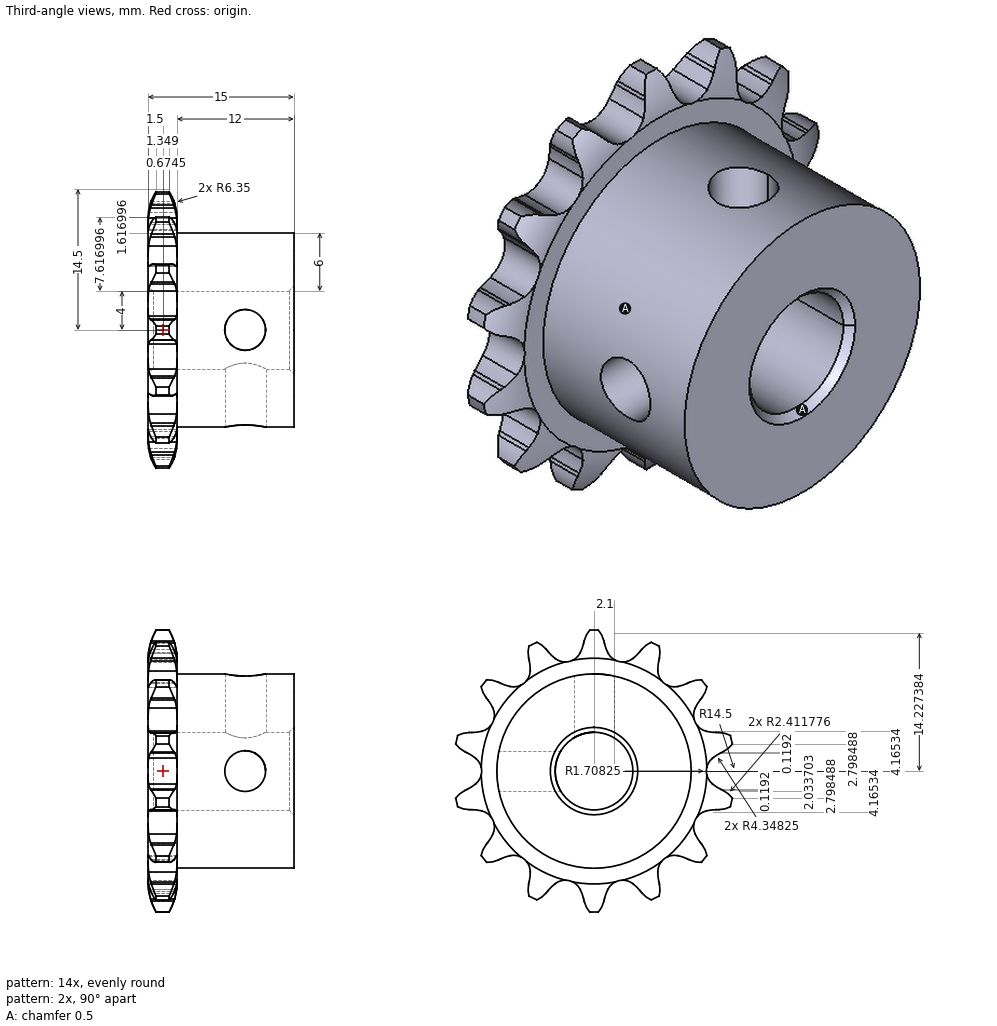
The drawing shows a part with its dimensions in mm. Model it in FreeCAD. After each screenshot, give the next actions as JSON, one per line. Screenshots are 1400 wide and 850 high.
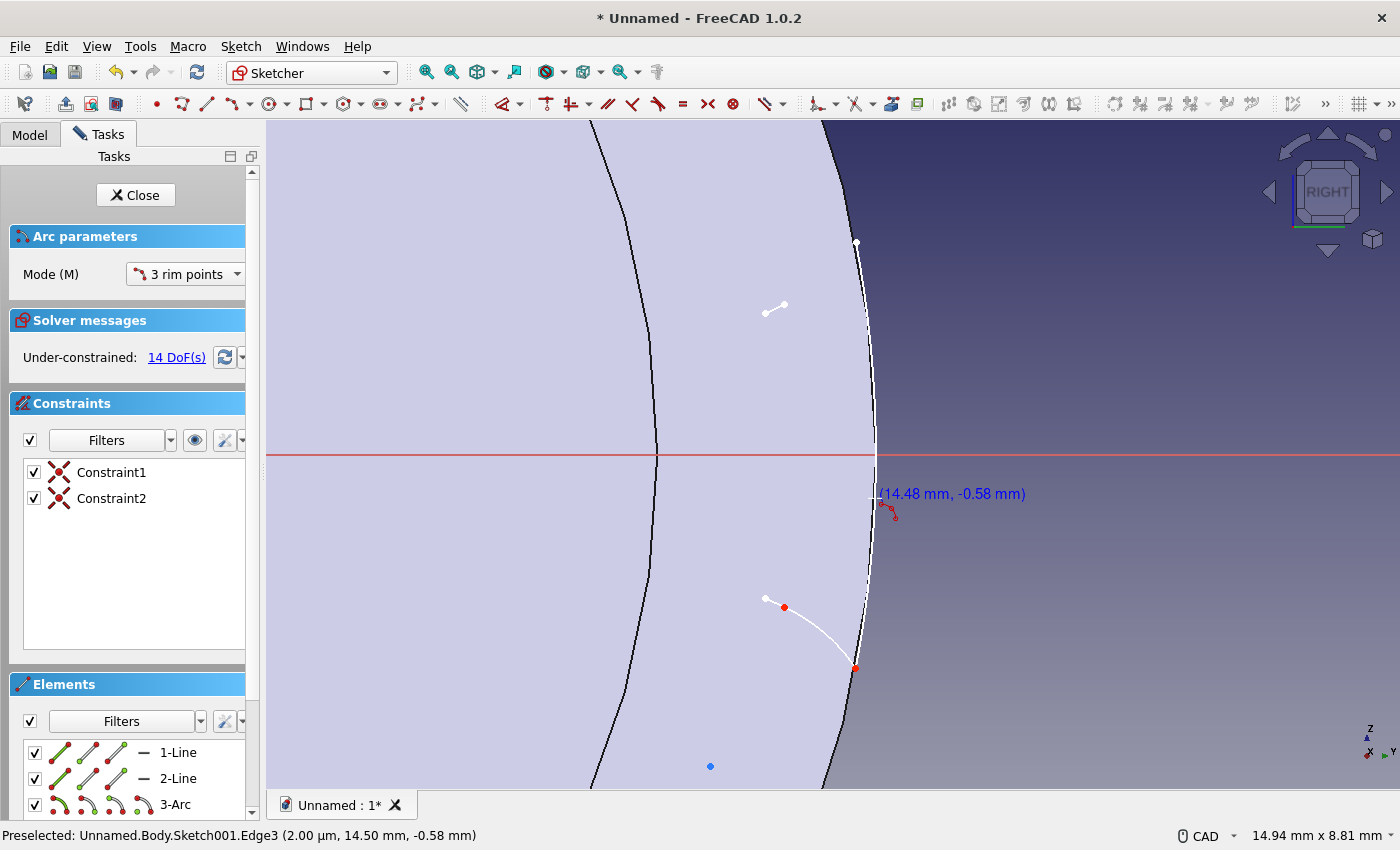
{"action": "left_click", "coordinate": [856, 243]}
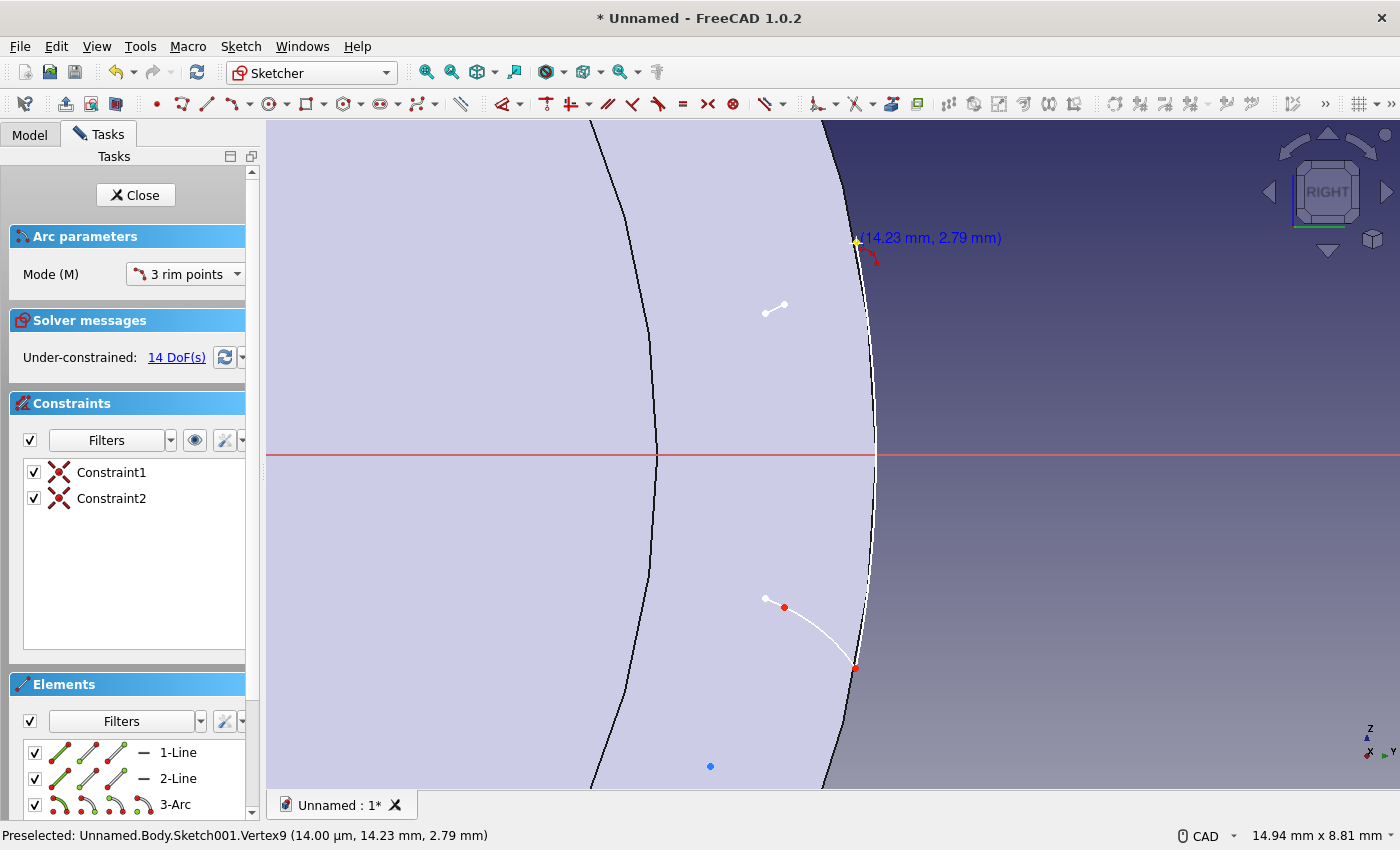
{"action": "scroll", "coordinate": [785, 303], "scroll_direction": "up", "scroll_amount": 3}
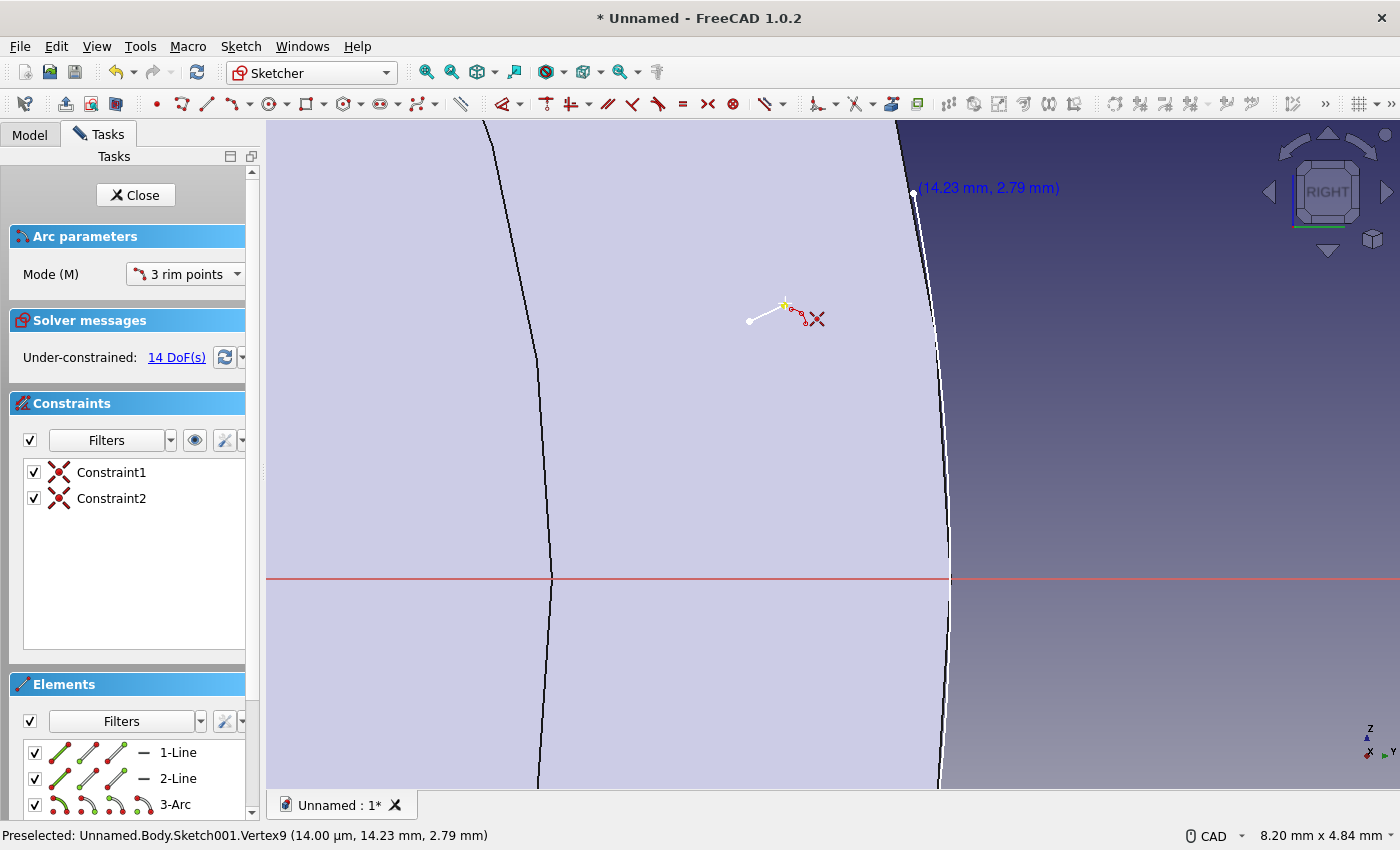
{"action": "left_click", "coordinate": [784, 305]}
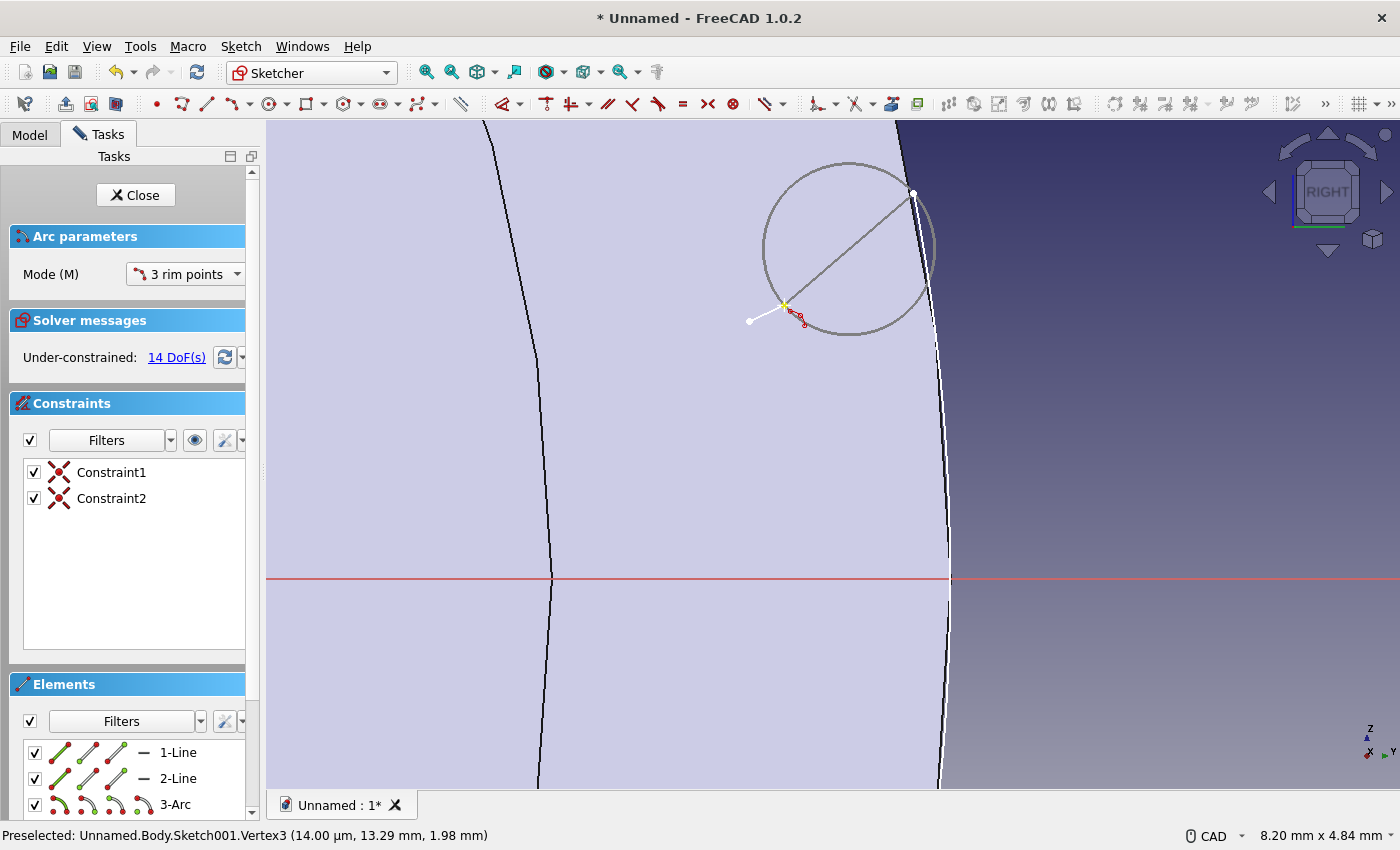
{"action": "scroll", "coordinate": [856, 256], "scroll_direction": "up", "scroll_amount": 2}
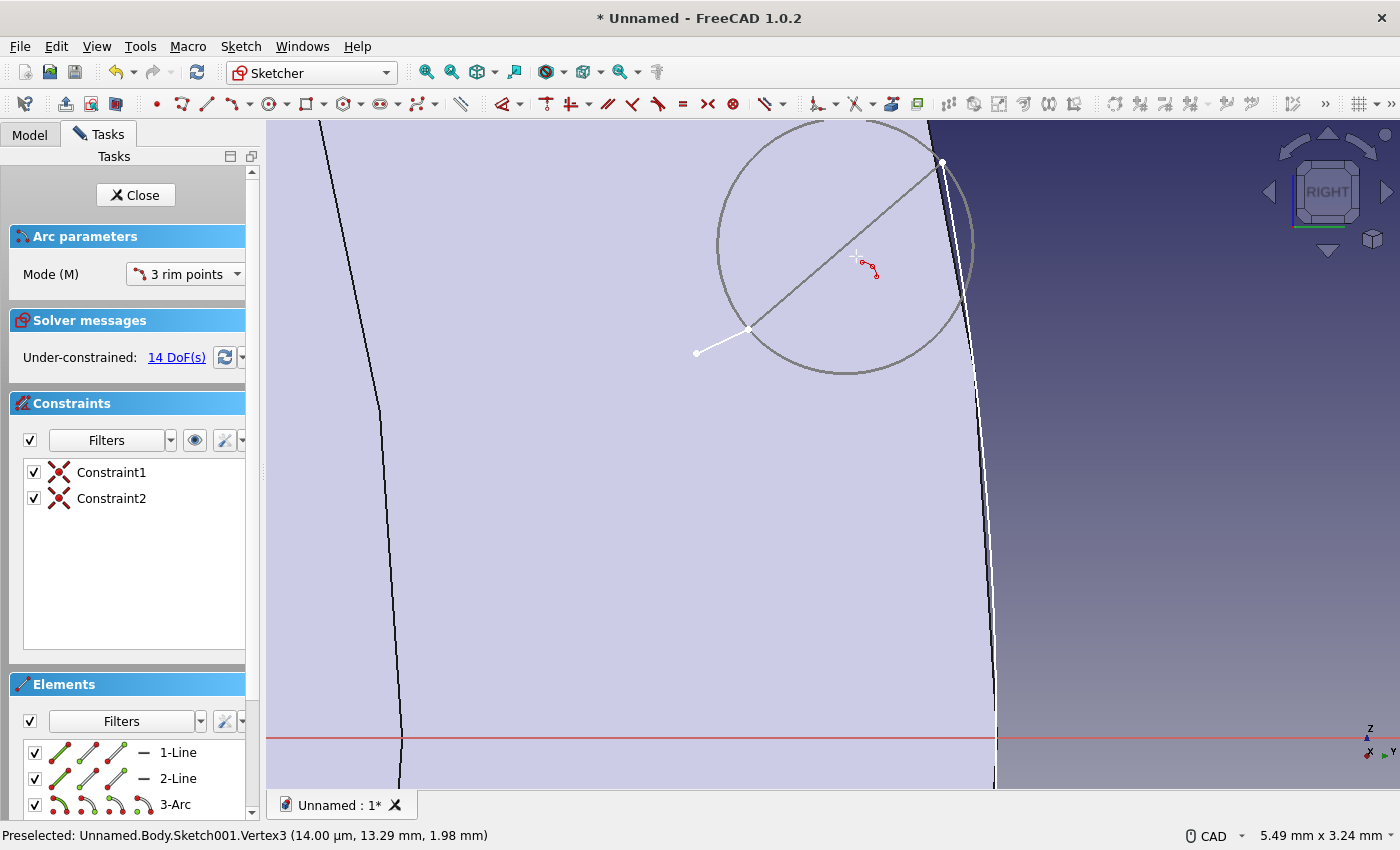
{"action": "left_click", "coordinate": [855, 256]}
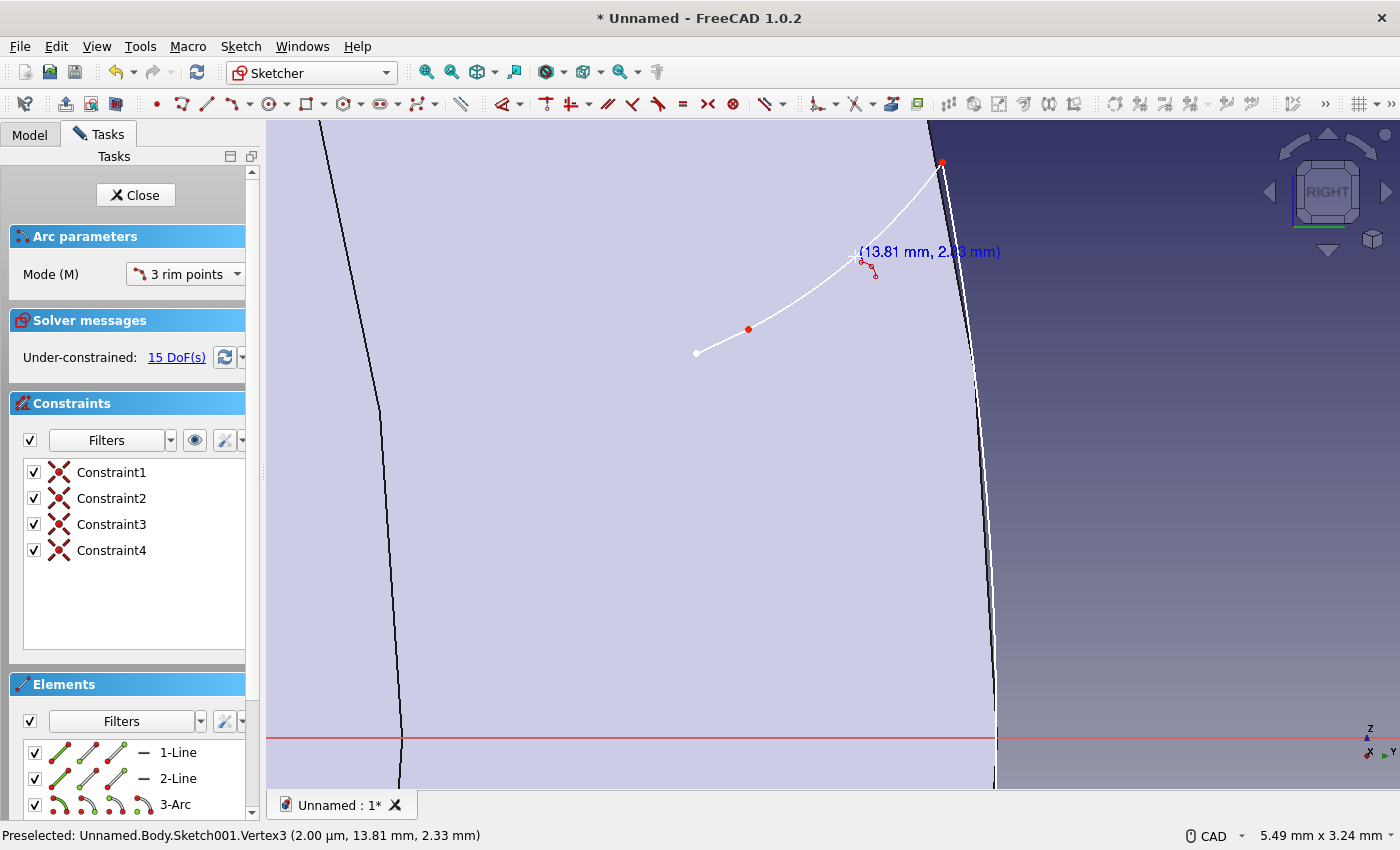
{"action": "left_click", "coordinate": [697, 354]}
{"action": "left_click", "coordinate": [518, 467]}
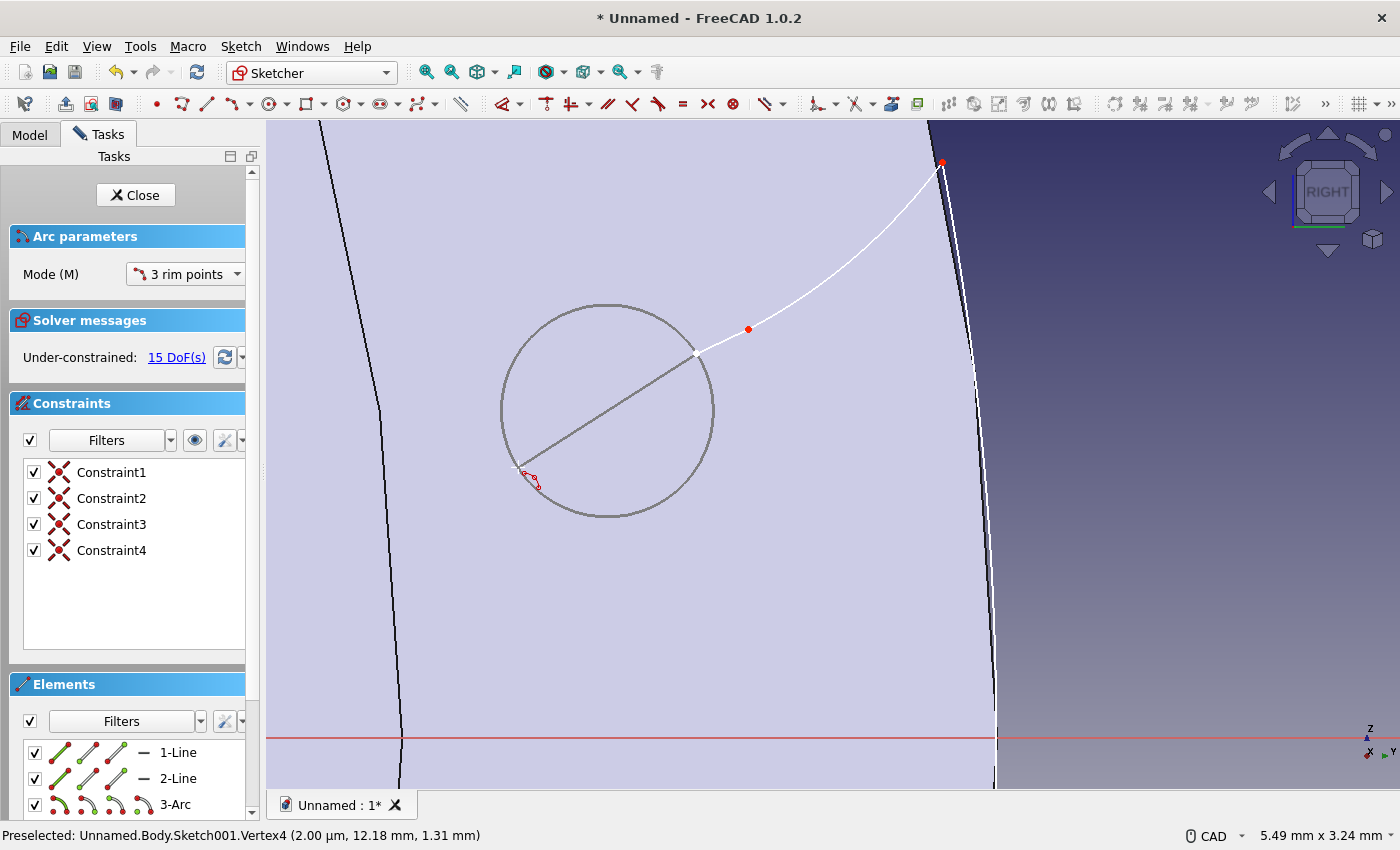
{"action": "scroll", "coordinate": [604, 404], "scroll_direction": "up", "scroll_amount": 5}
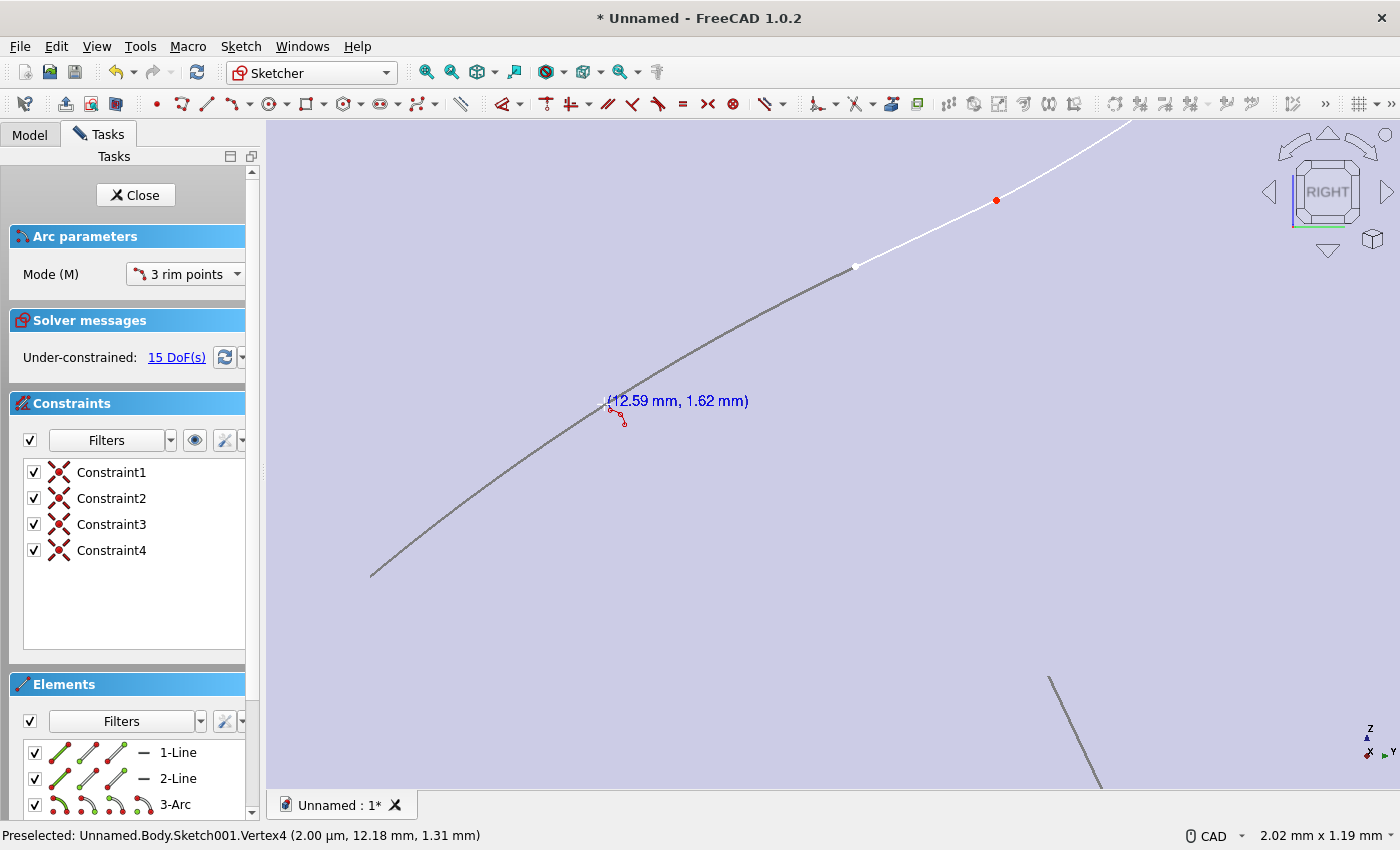
{"action": "left_click", "coordinate": [605, 402]}